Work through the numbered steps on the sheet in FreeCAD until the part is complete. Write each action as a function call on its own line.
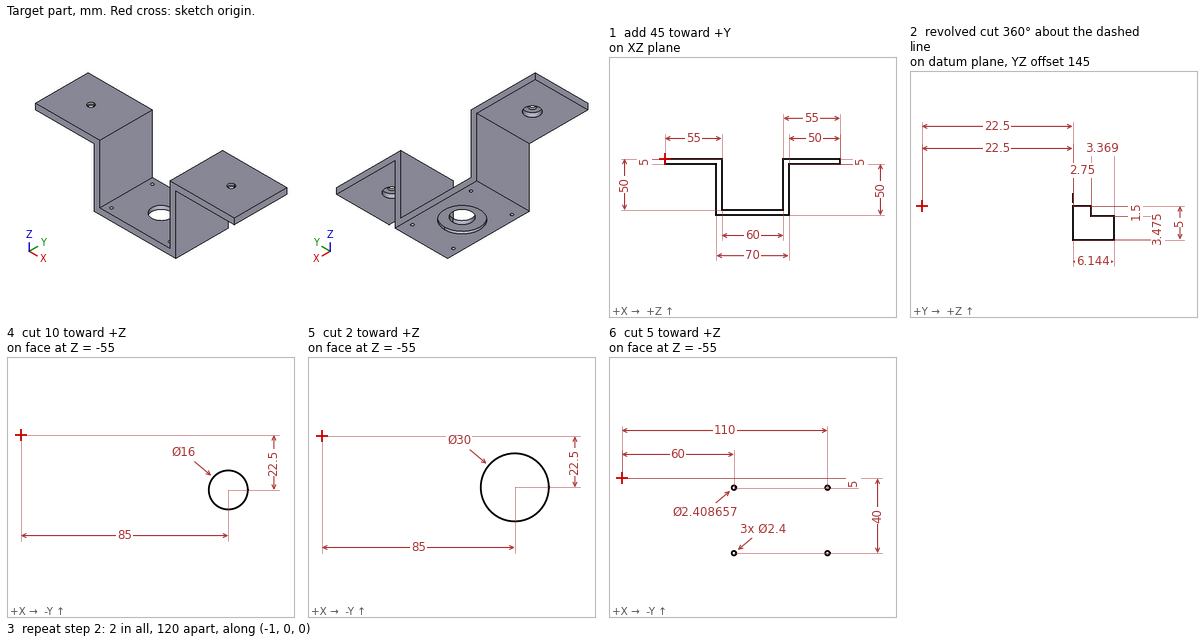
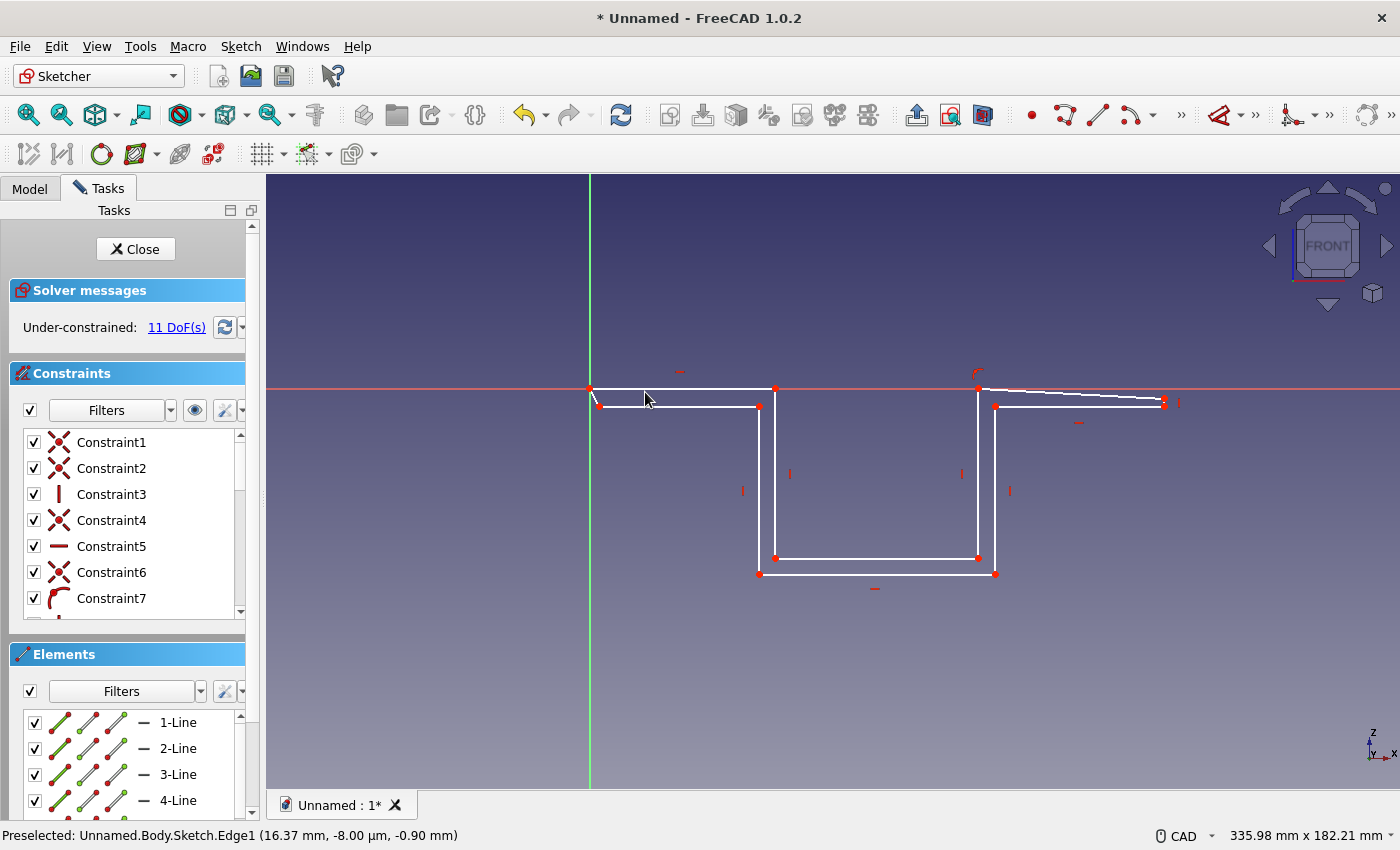
click(1034, 392)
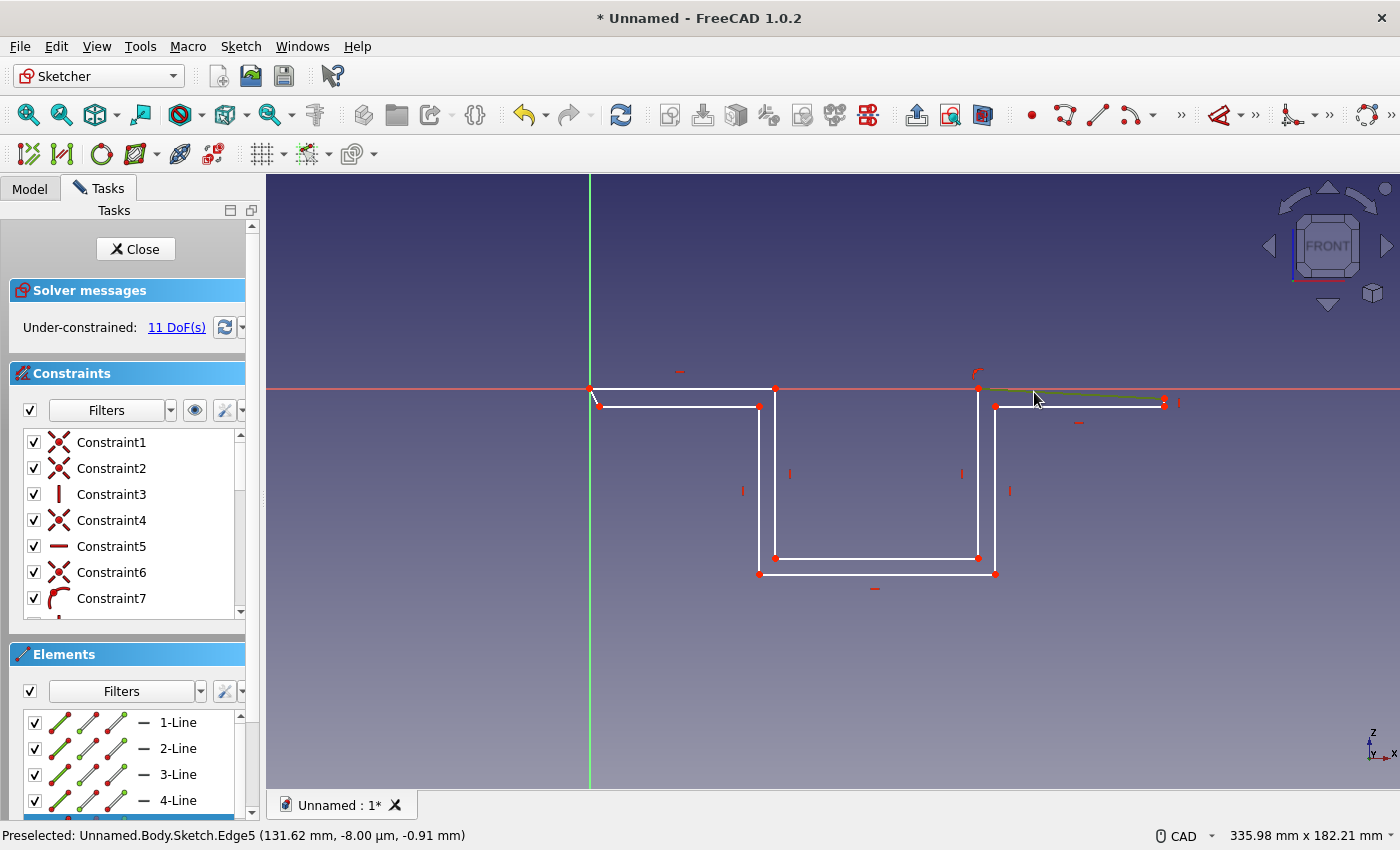
key(h)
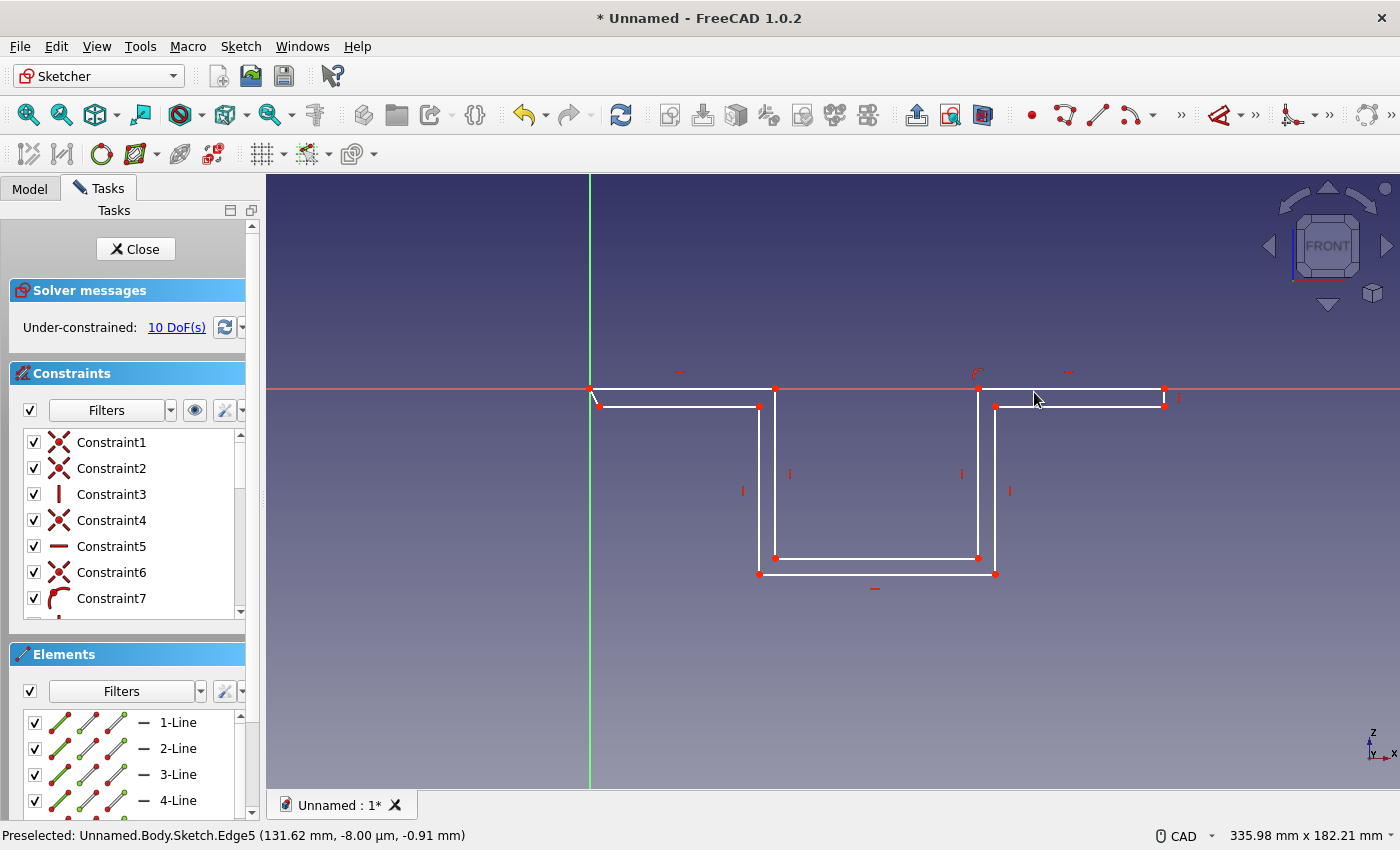
scroll(593, 396, up, 4)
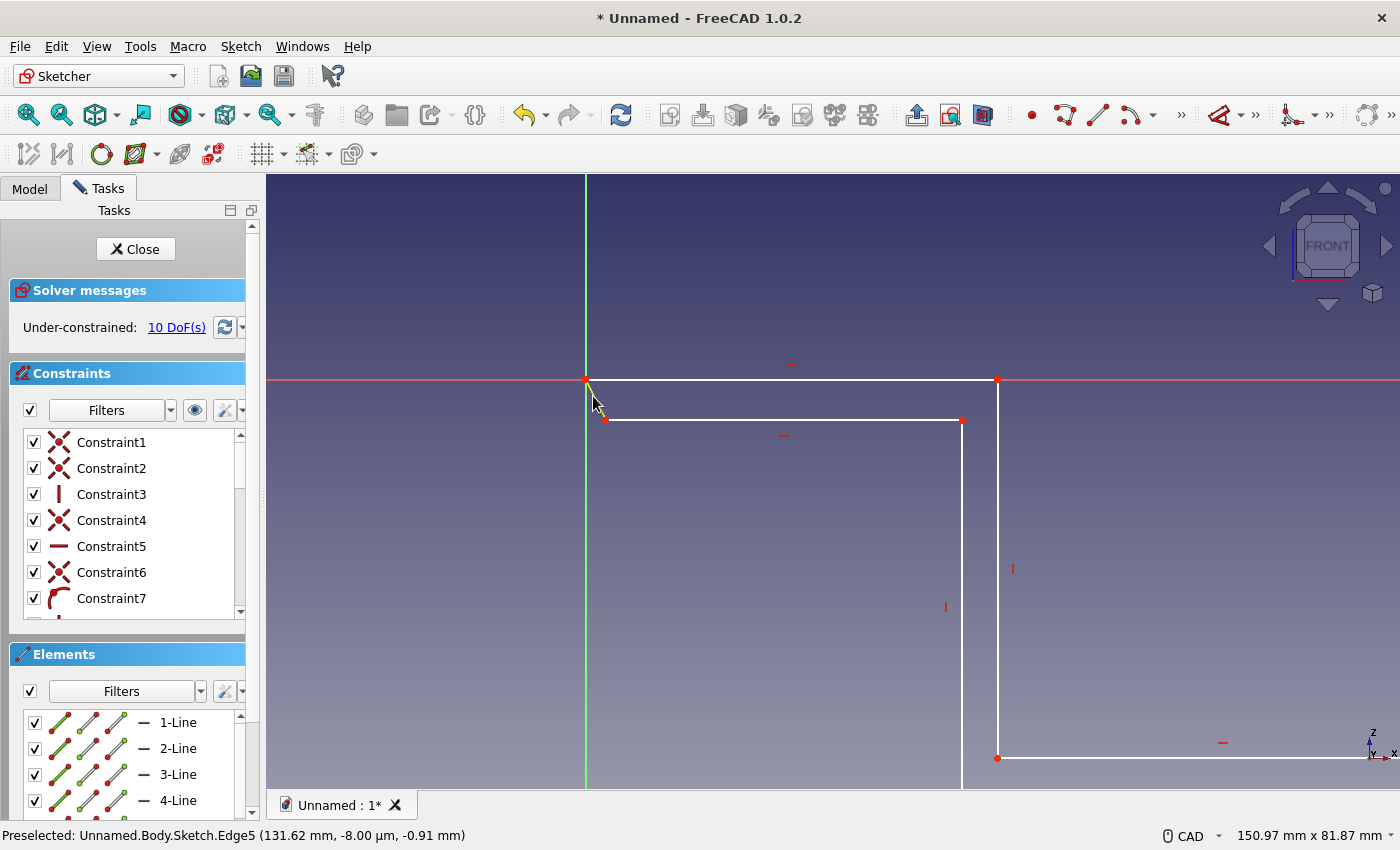
click(594, 396)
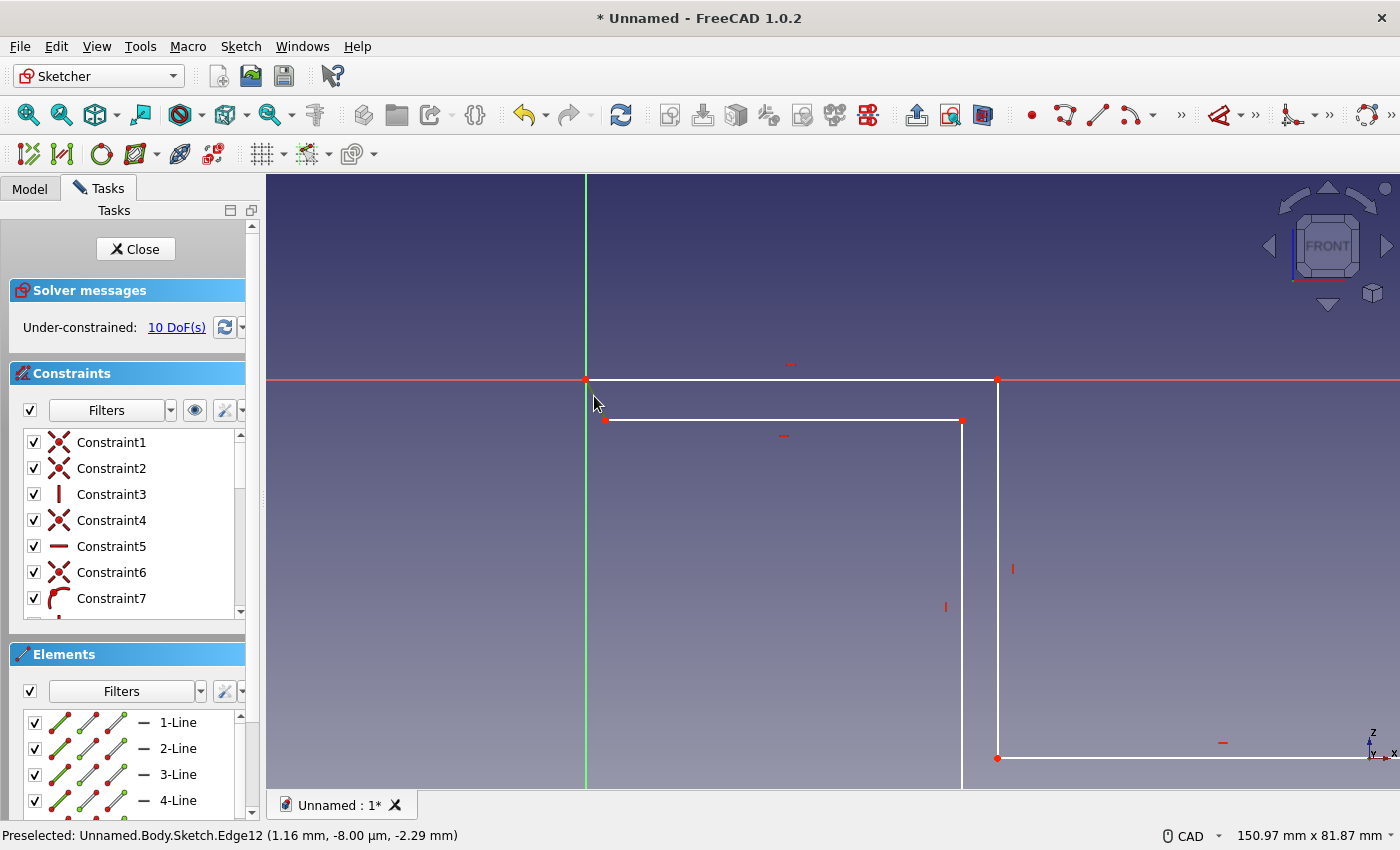
key(v)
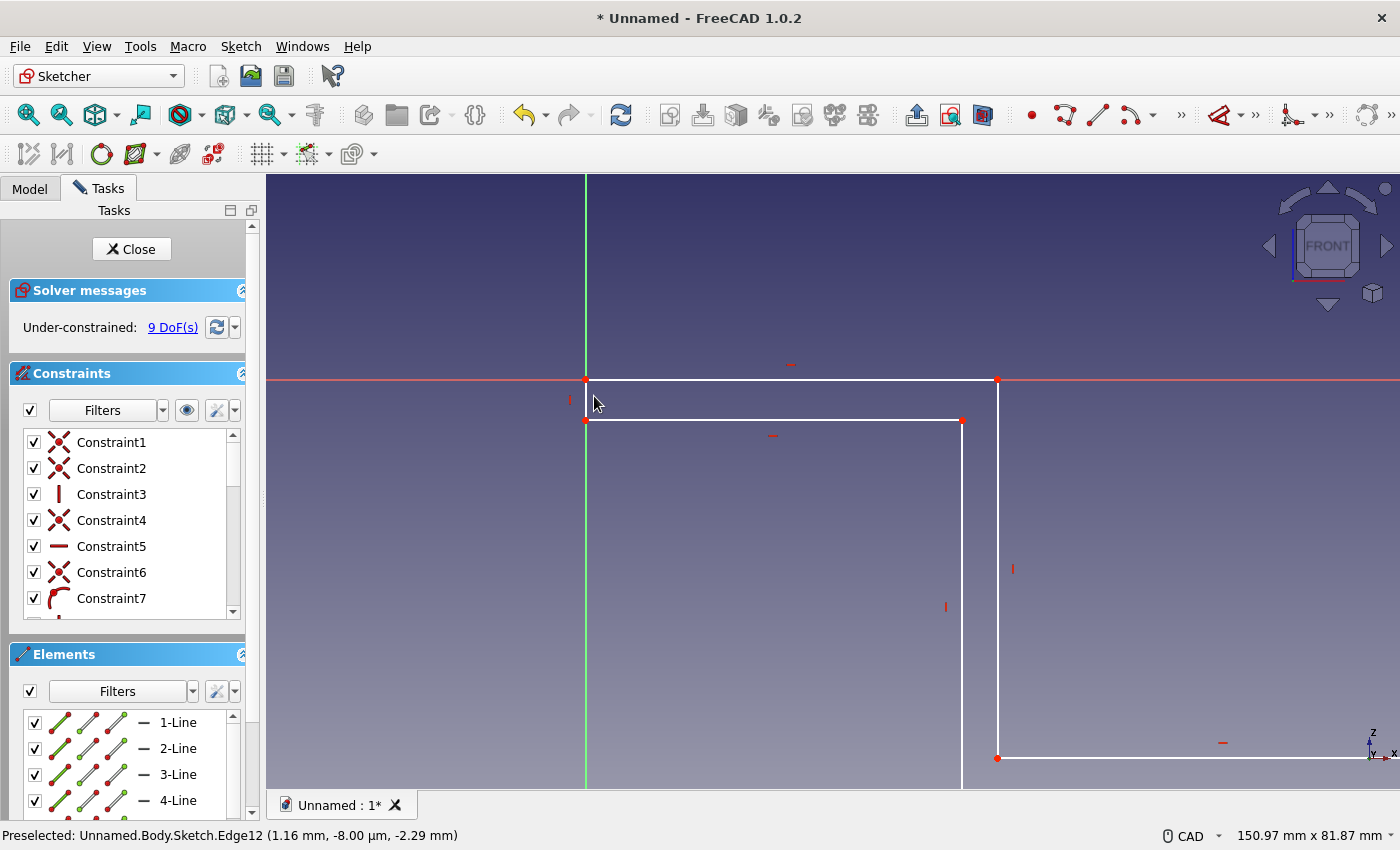
click(1218, 116)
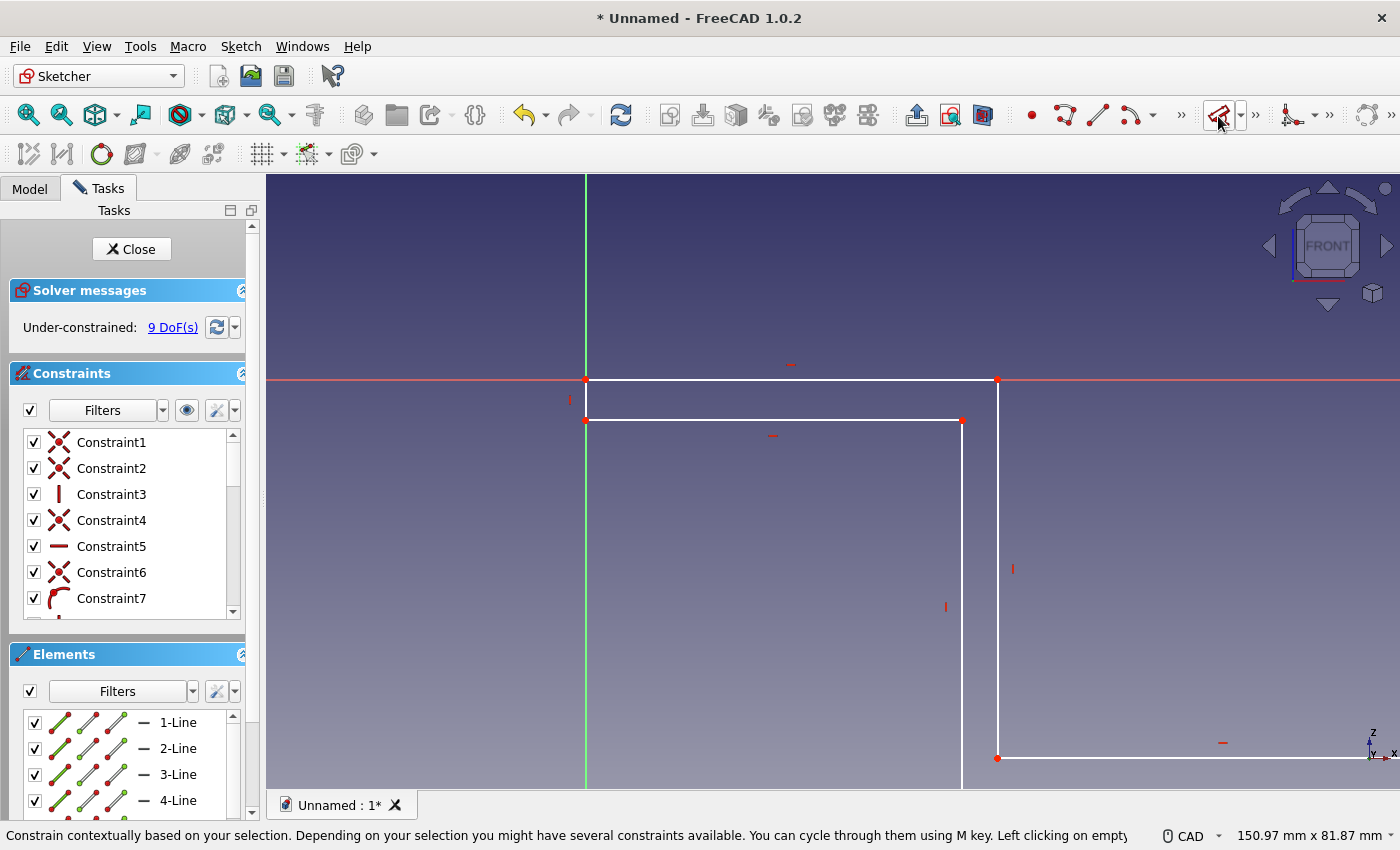
scroll(294, 354, down, 3)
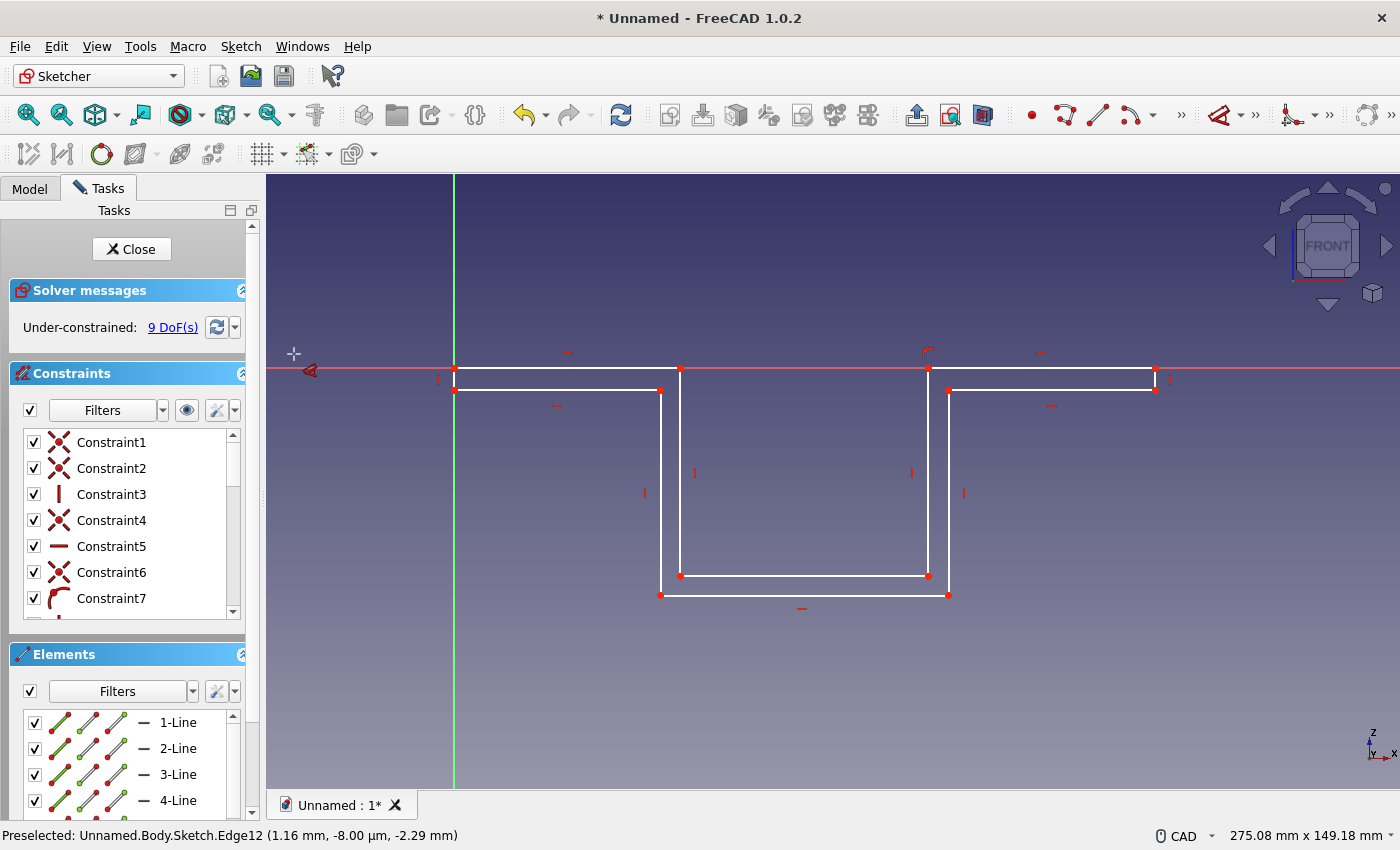
scroll(1155, 375, up, 4)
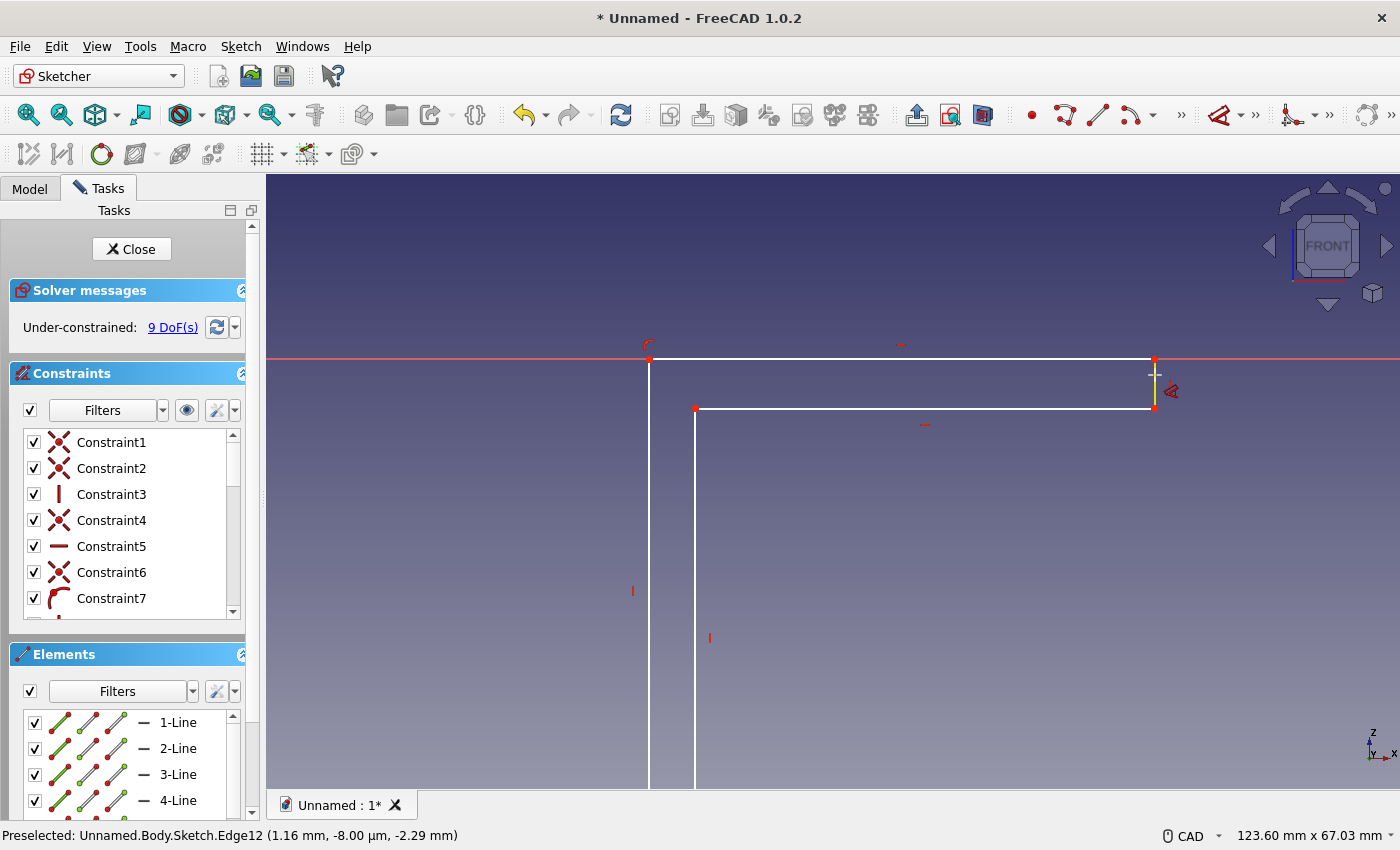
click(1155, 374)
click(1189, 384)